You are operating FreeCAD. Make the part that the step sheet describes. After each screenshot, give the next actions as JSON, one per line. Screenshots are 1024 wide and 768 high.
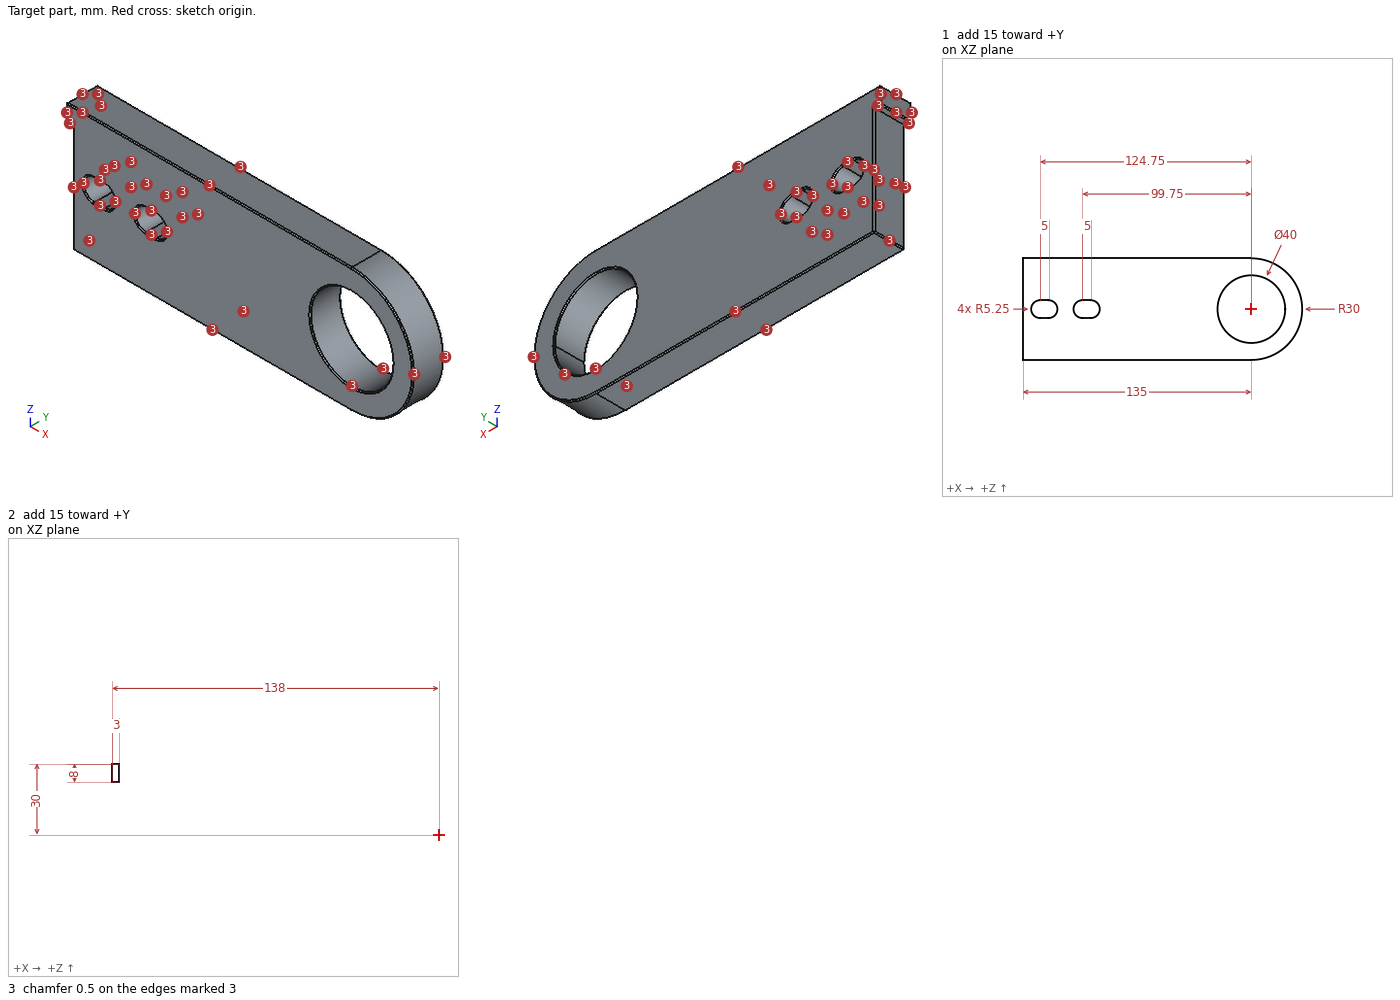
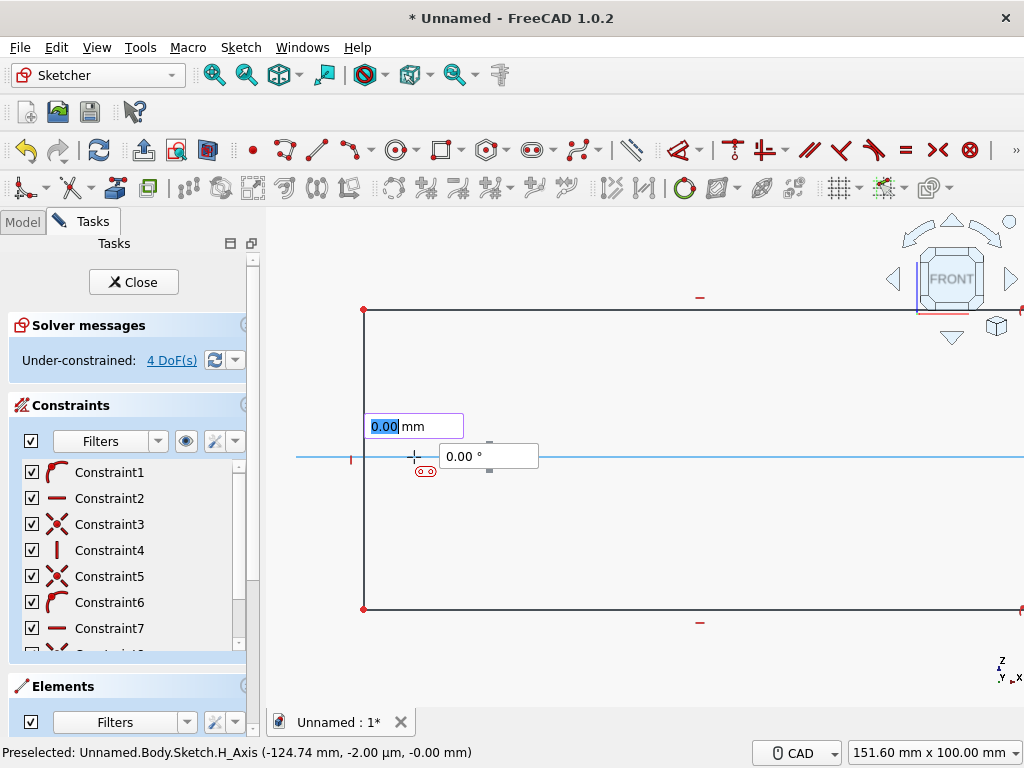
{"action": "left_click", "coordinate": [439, 448]}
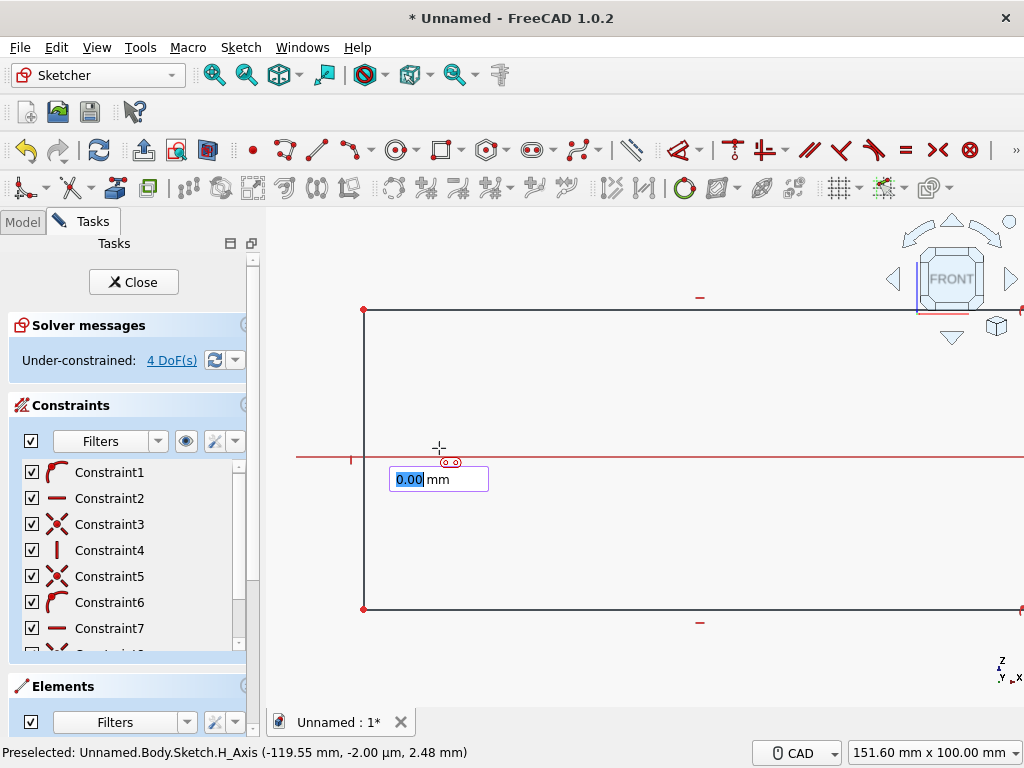
{"action": "left_click", "coordinate": [426, 483]}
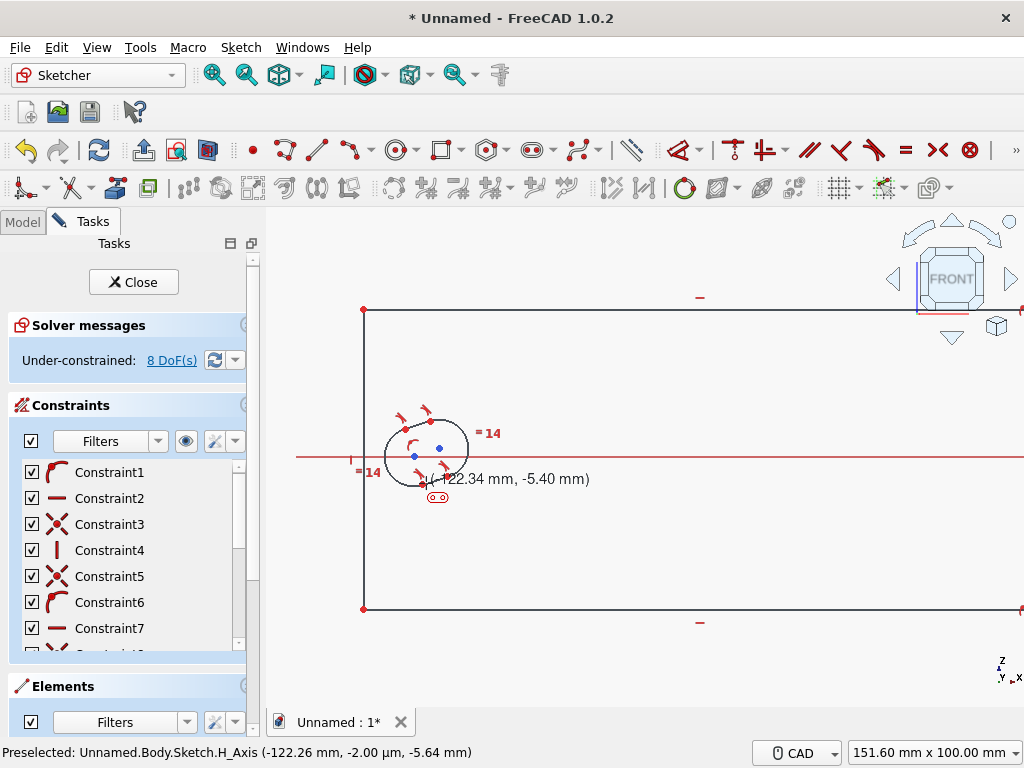
{"action": "left_click", "coordinate": [539, 457]}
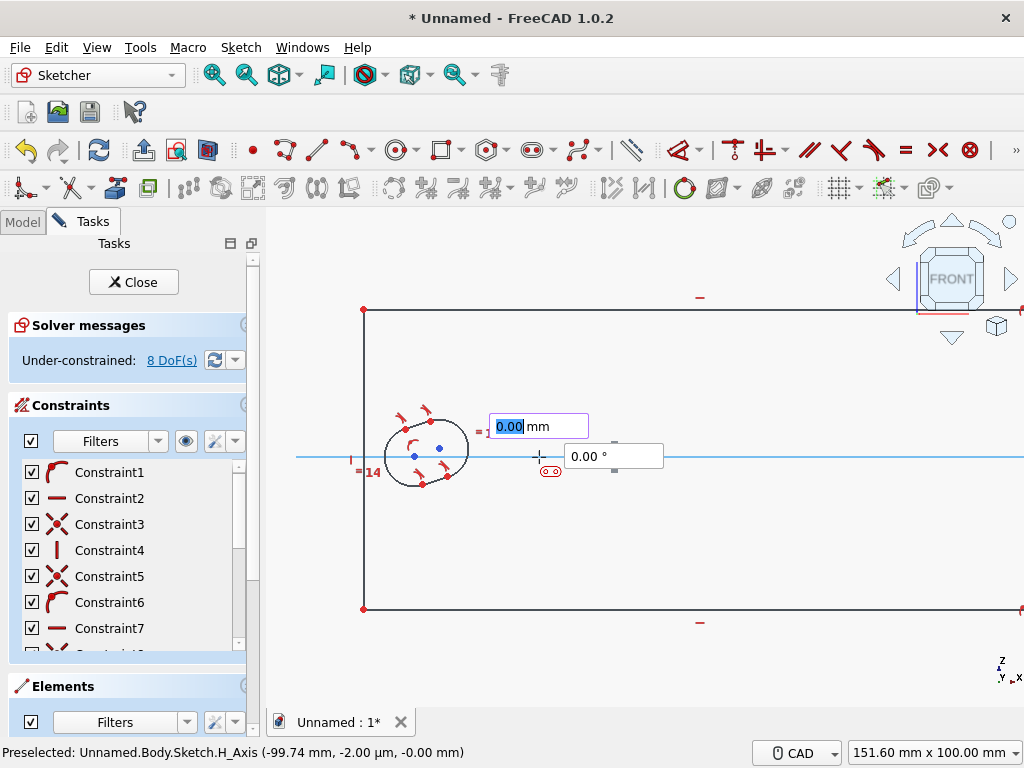
{"action": "left_click", "coordinate": [564, 448]}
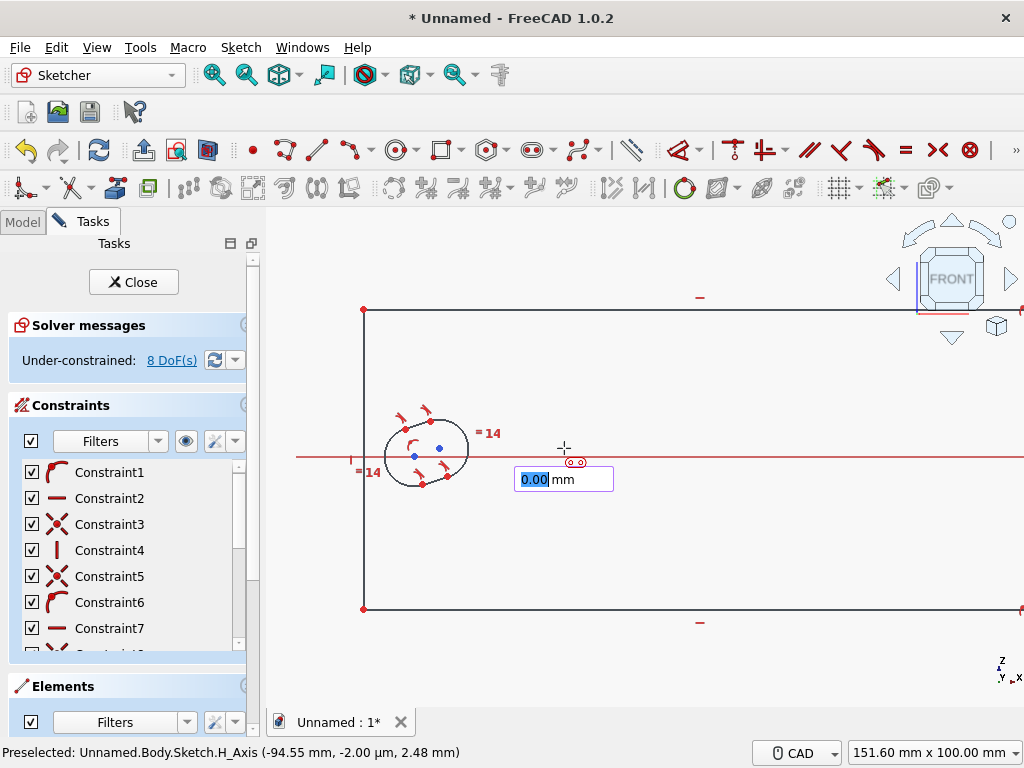
{"action": "left_click", "coordinate": [551, 483]}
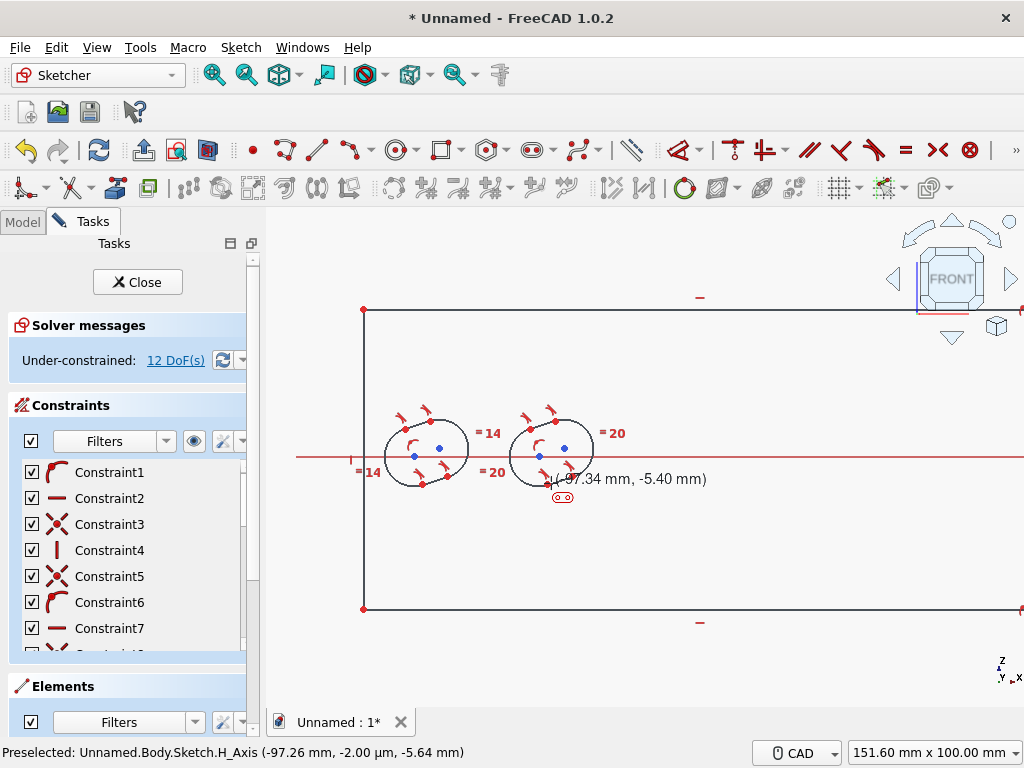
{"action": "left_click", "coordinate": [396, 150]}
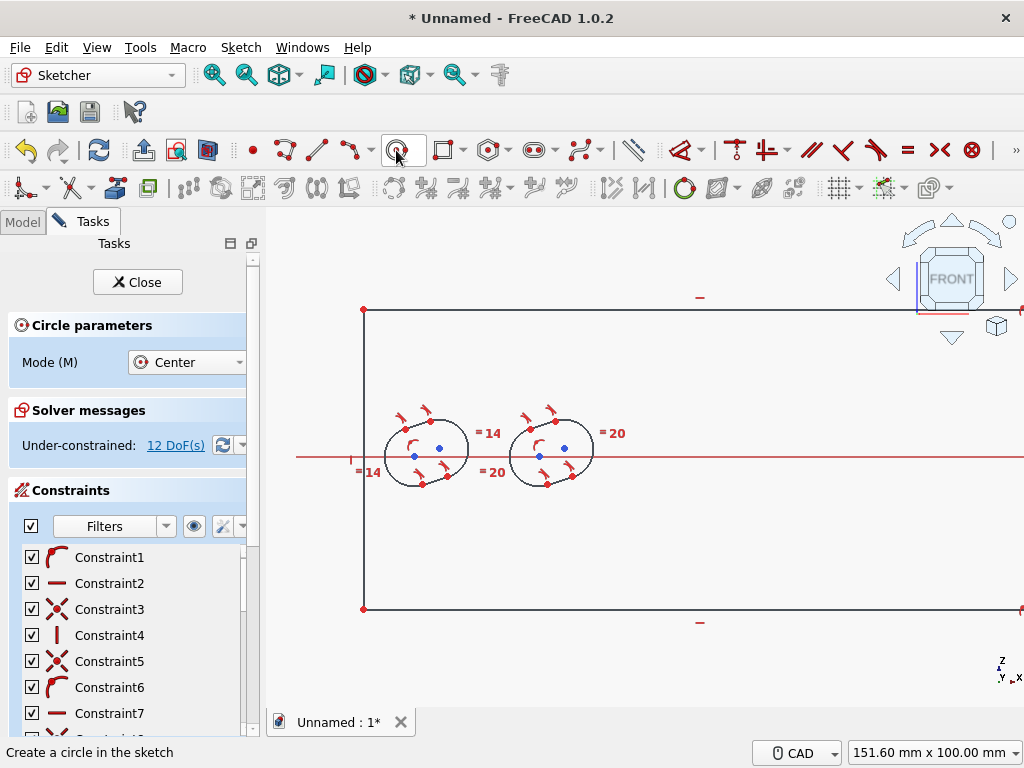
{"action": "scroll", "coordinate": [414, 457], "scroll_direction": "down", "scroll_amount": 4}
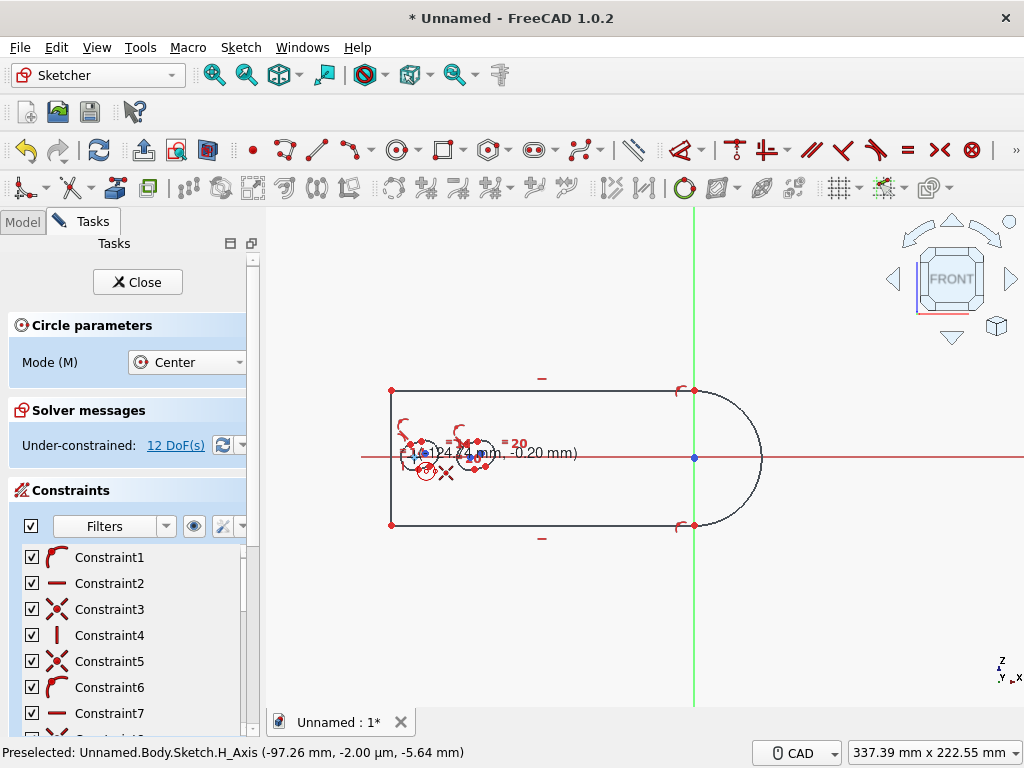
{"action": "left_click", "coordinate": [694, 457]}
{"action": "mouse_move", "coordinate": [726, 426]}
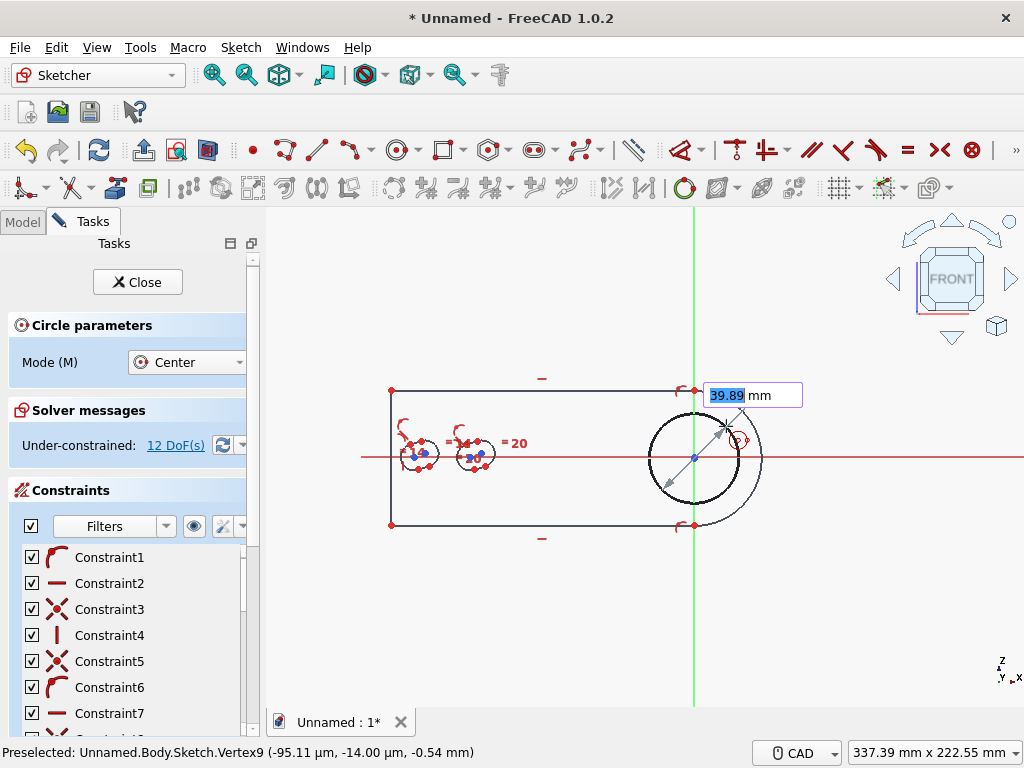
{"action": "type", "text": "40"}
{"action": "key", "text": "Return"}
{"action": "key", "text": "Escape"}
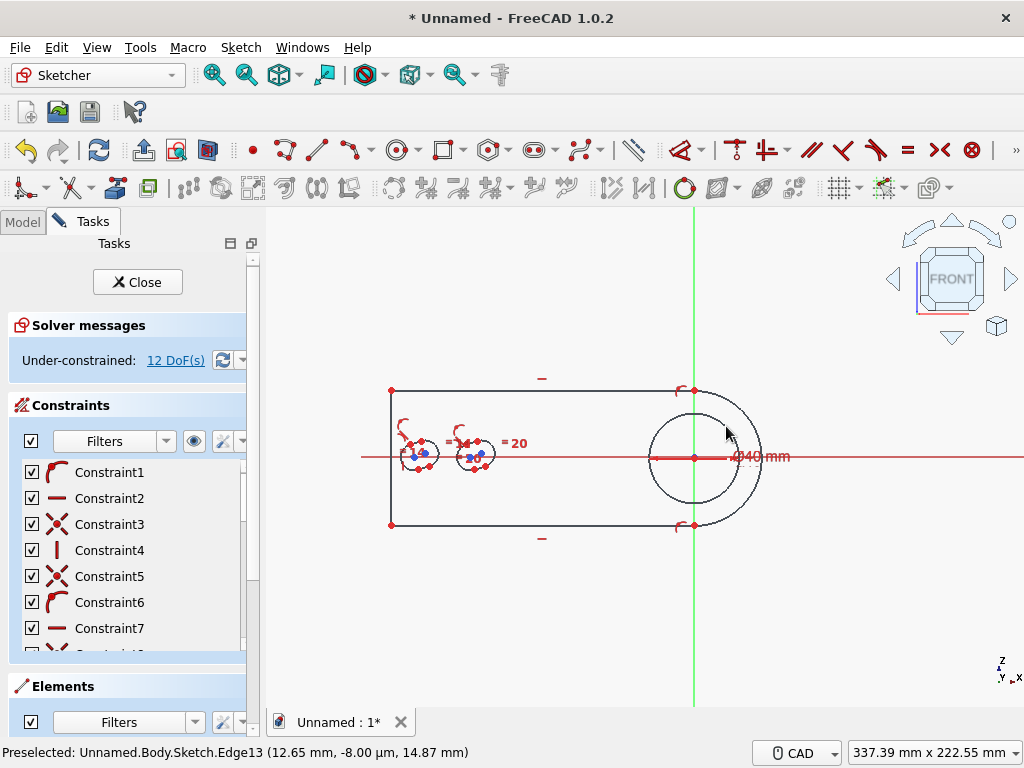
{"action": "scroll", "coordinate": [416, 443], "scroll_direction": "up", "scroll_amount": 5}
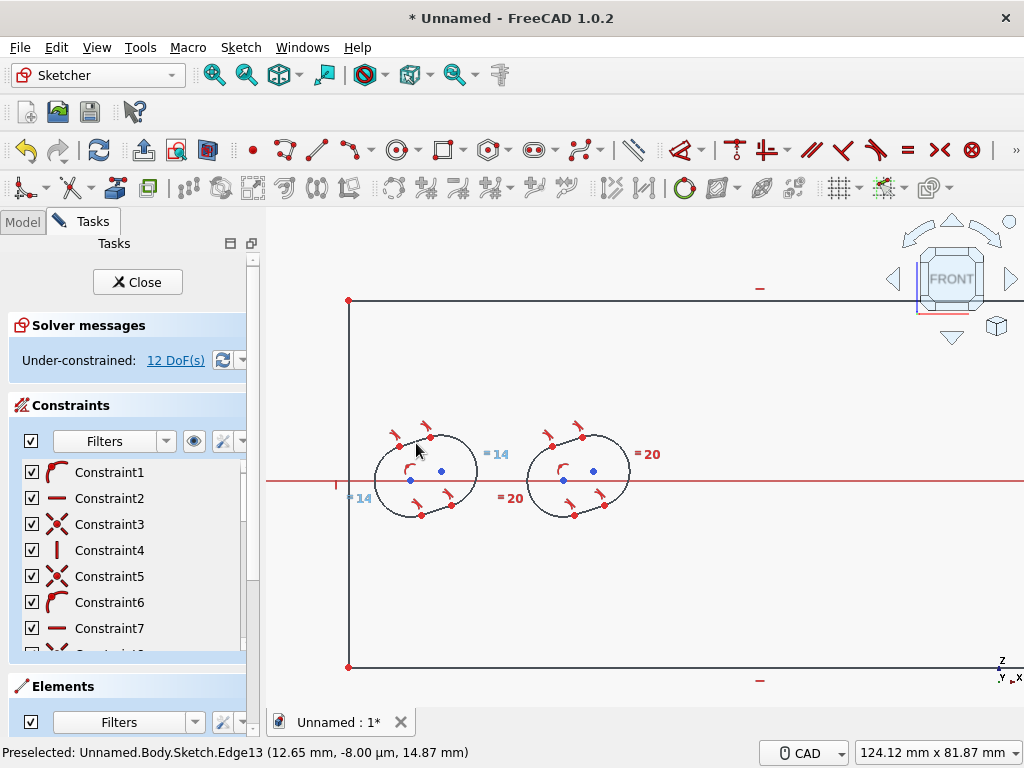
{"action": "left_click", "coordinate": [415, 442]}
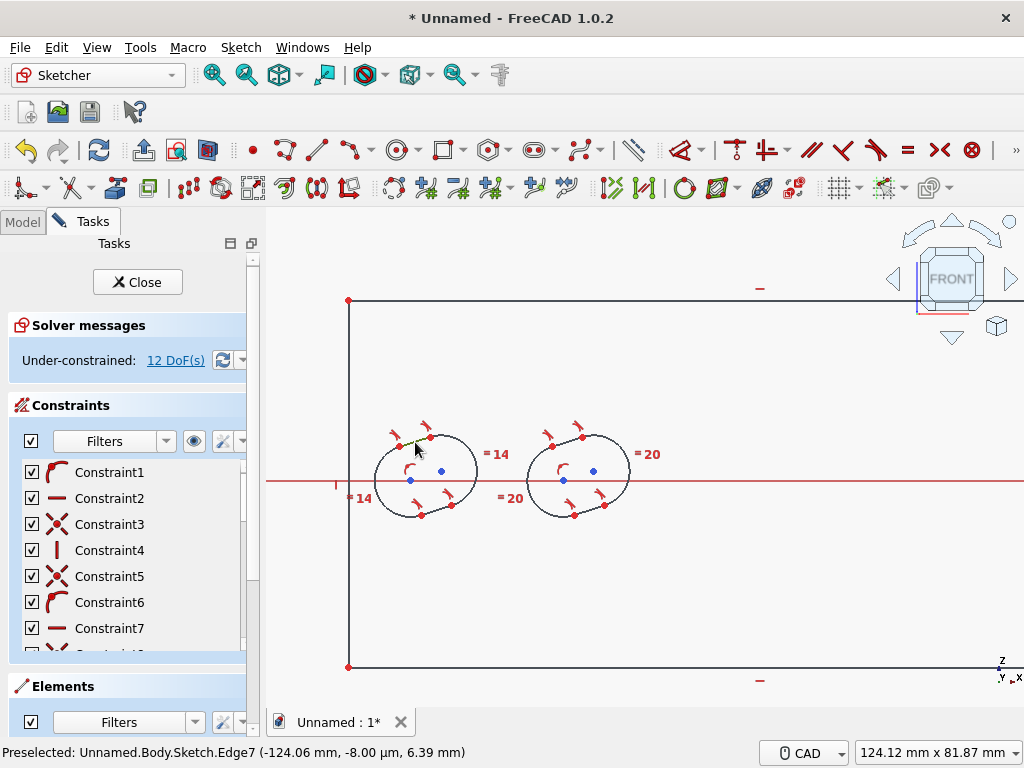
{"action": "left_click", "coordinate": [790, 150]}